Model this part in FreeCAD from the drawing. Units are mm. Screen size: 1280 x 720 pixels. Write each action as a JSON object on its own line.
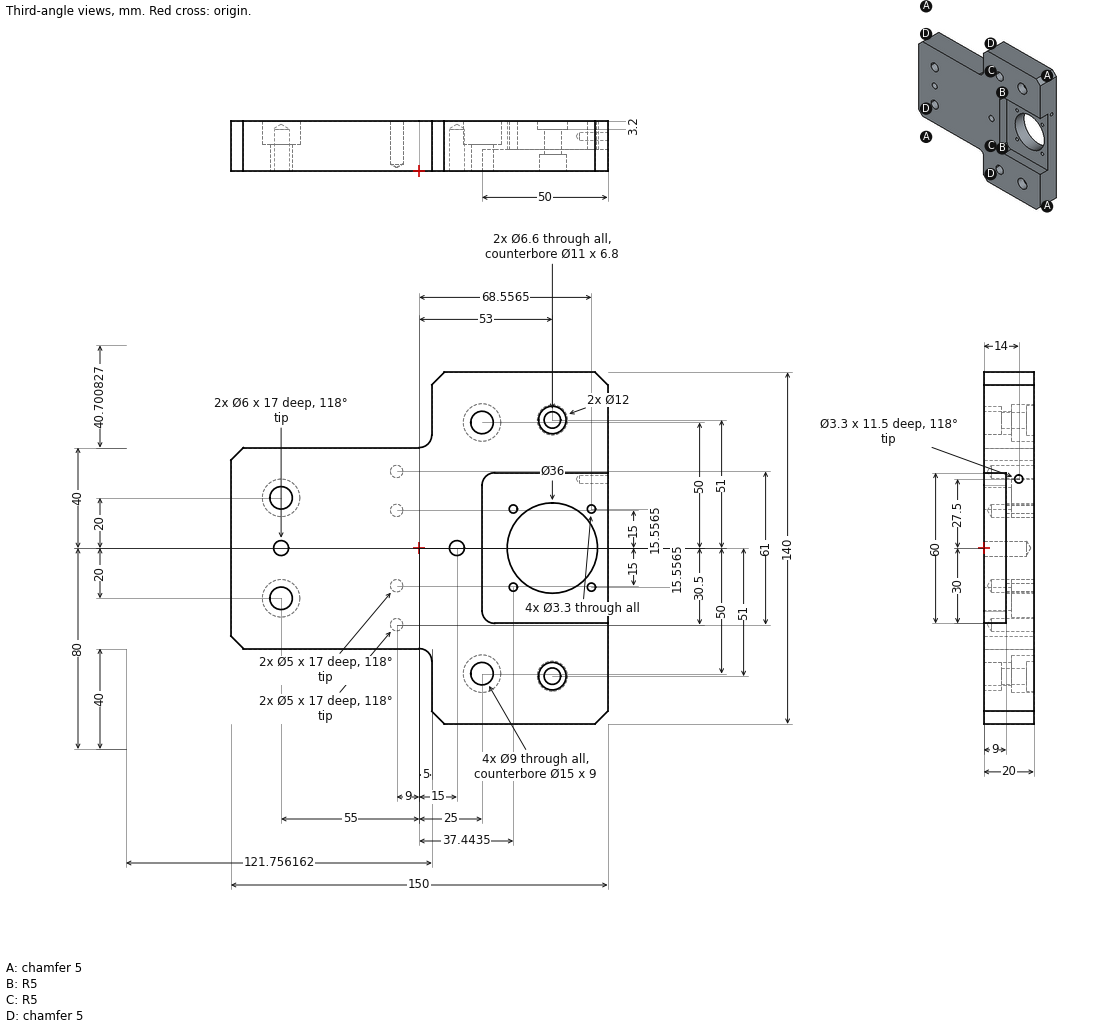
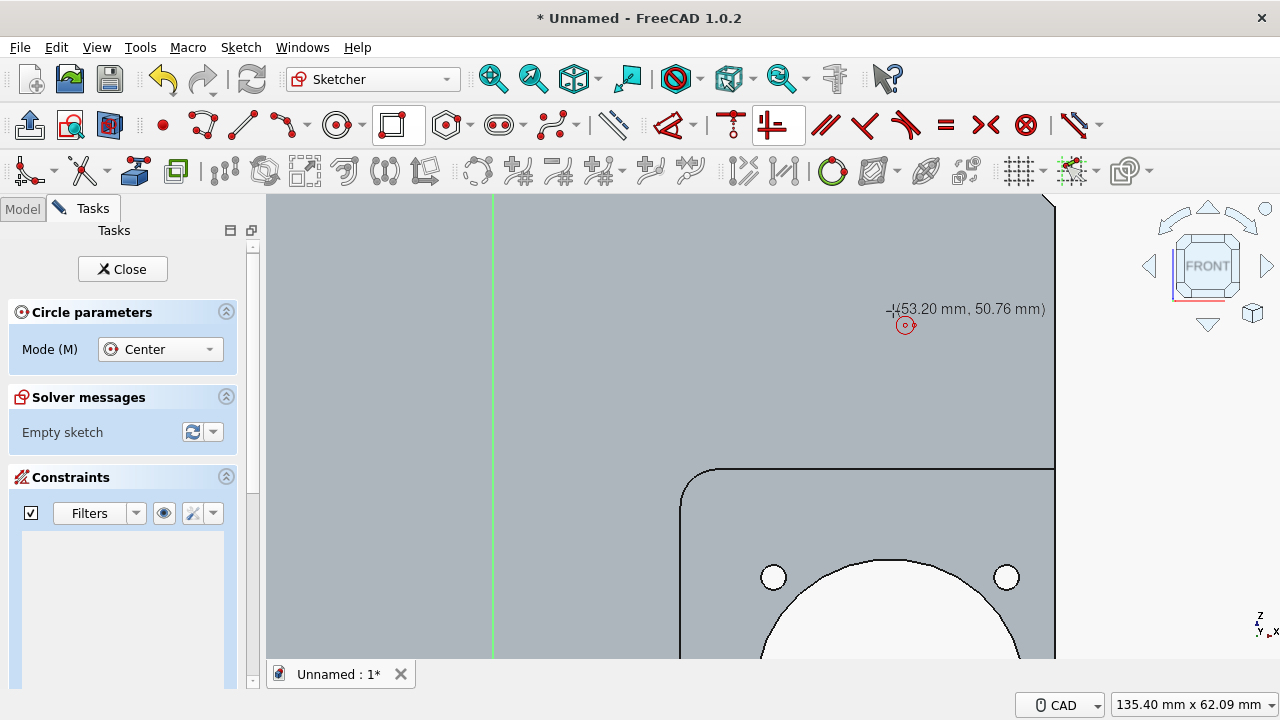
{"action": "left_click", "coordinate": [890, 312]}
{"action": "left_click", "coordinate": [908, 294]}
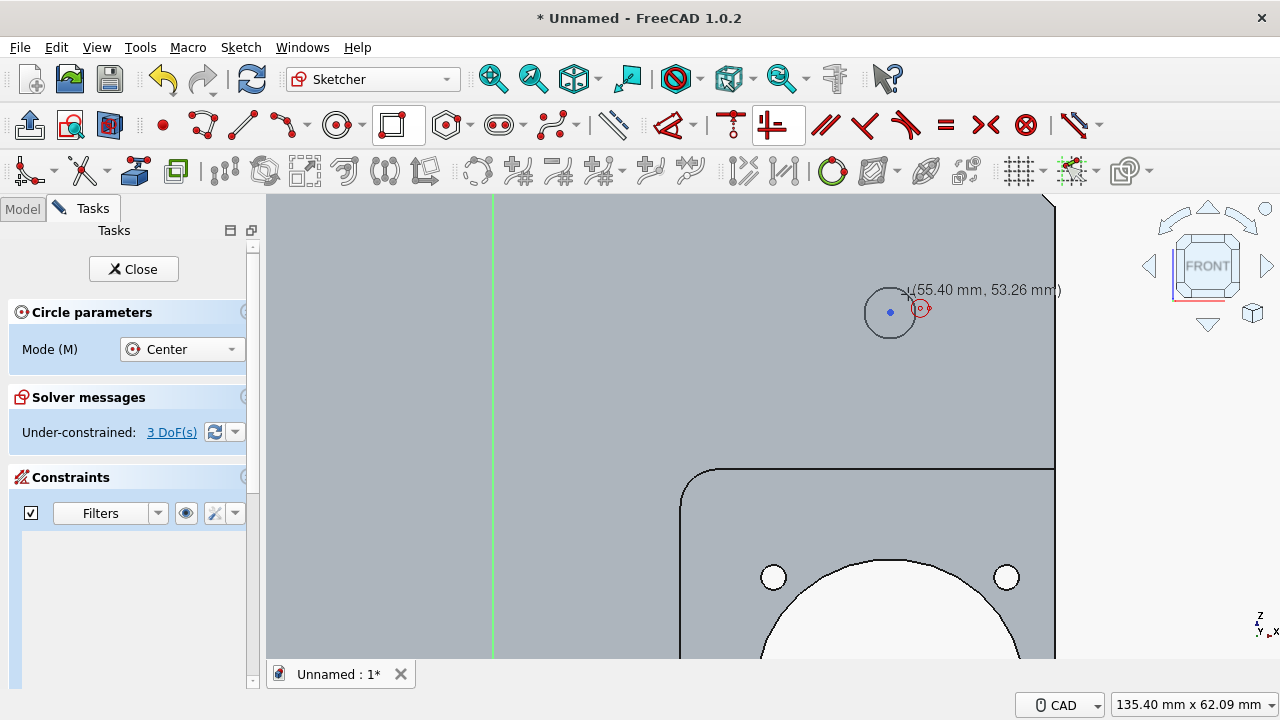
{"action": "scroll", "coordinate": [705, 271], "scroll_direction": "down", "scroll_amount": 5}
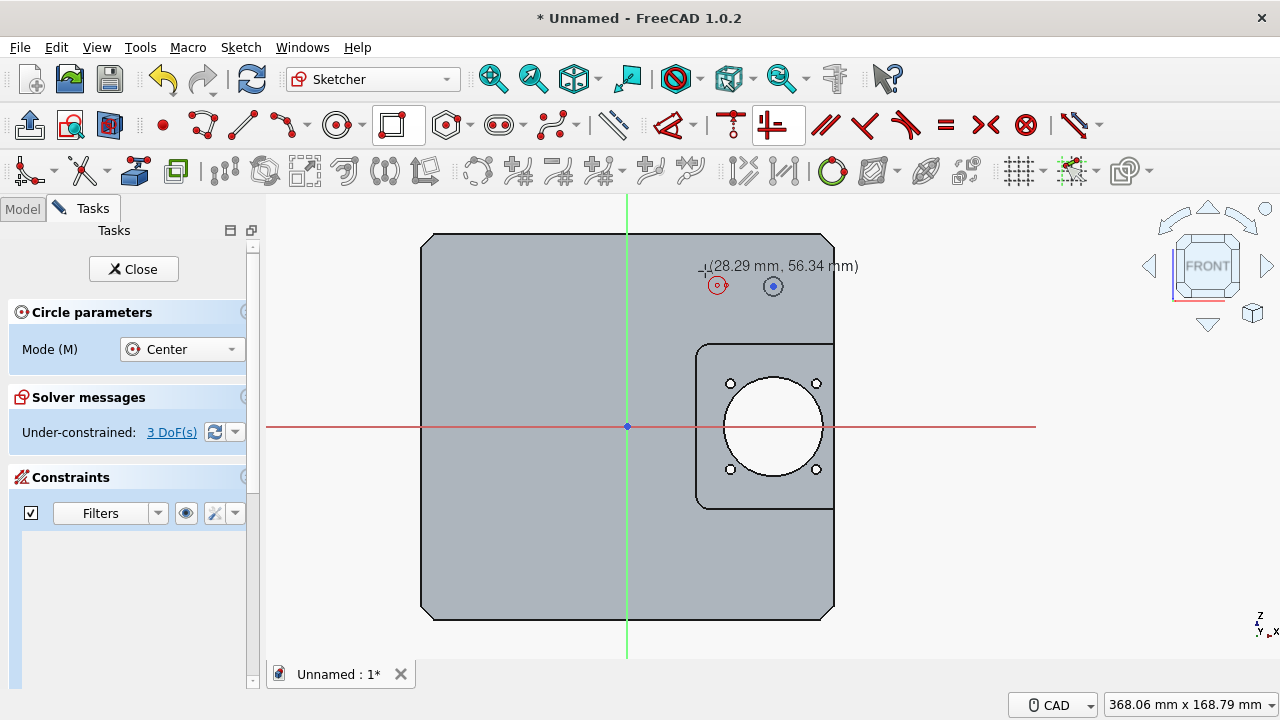
{"action": "scroll", "coordinate": [773, 567], "scroll_direction": "up", "scroll_amount": 5}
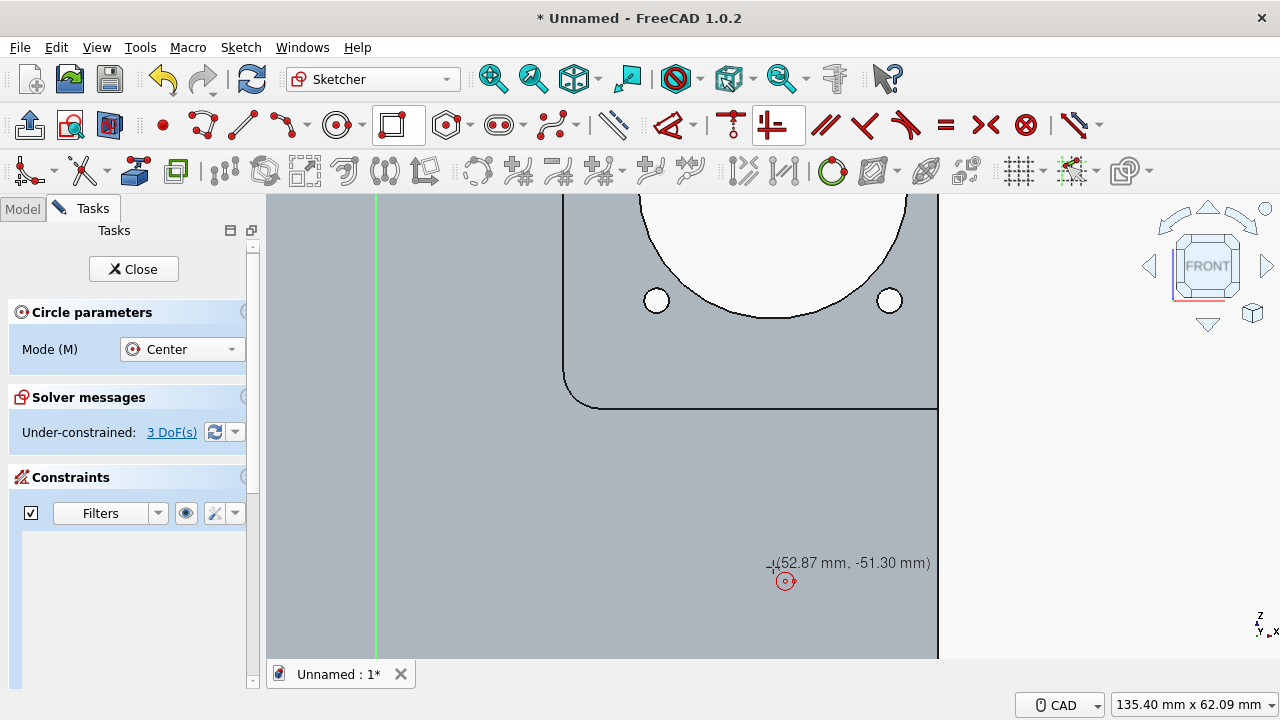
{"action": "left_click", "coordinate": [773, 566]}
{"action": "left_click", "coordinate": [791, 549]}
{"action": "key", "text": "Escape"}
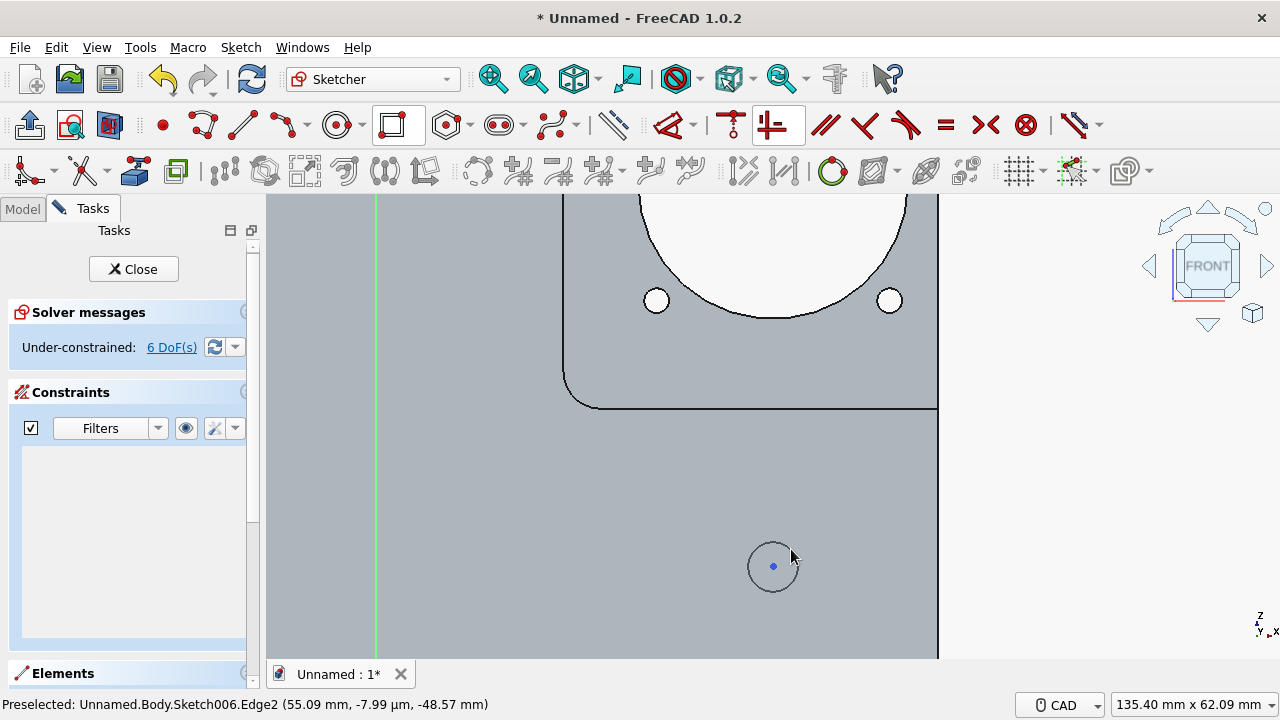
{"action": "scroll", "coordinate": [773, 568], "scroll_direction": "down", "scroll_amount": 5}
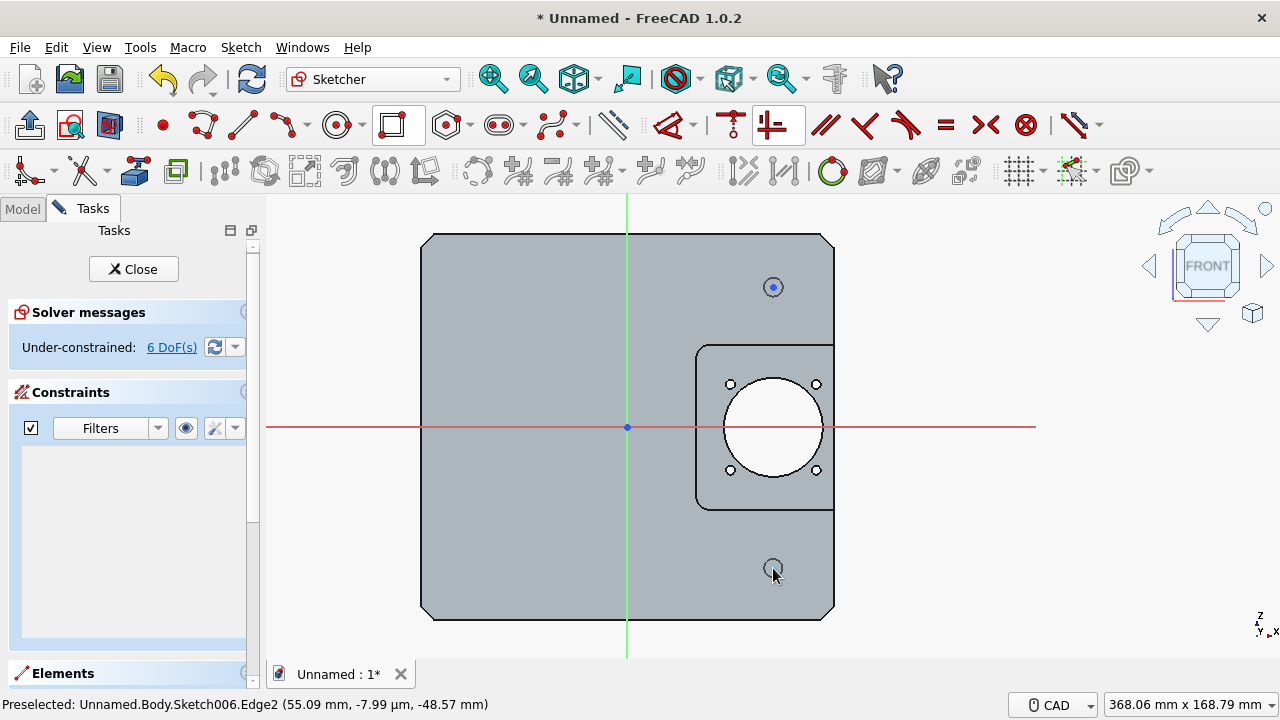
{"action": "scroll", "coordinate": [780, 281], "scroll_direction": "up", "scroll_amount": 2}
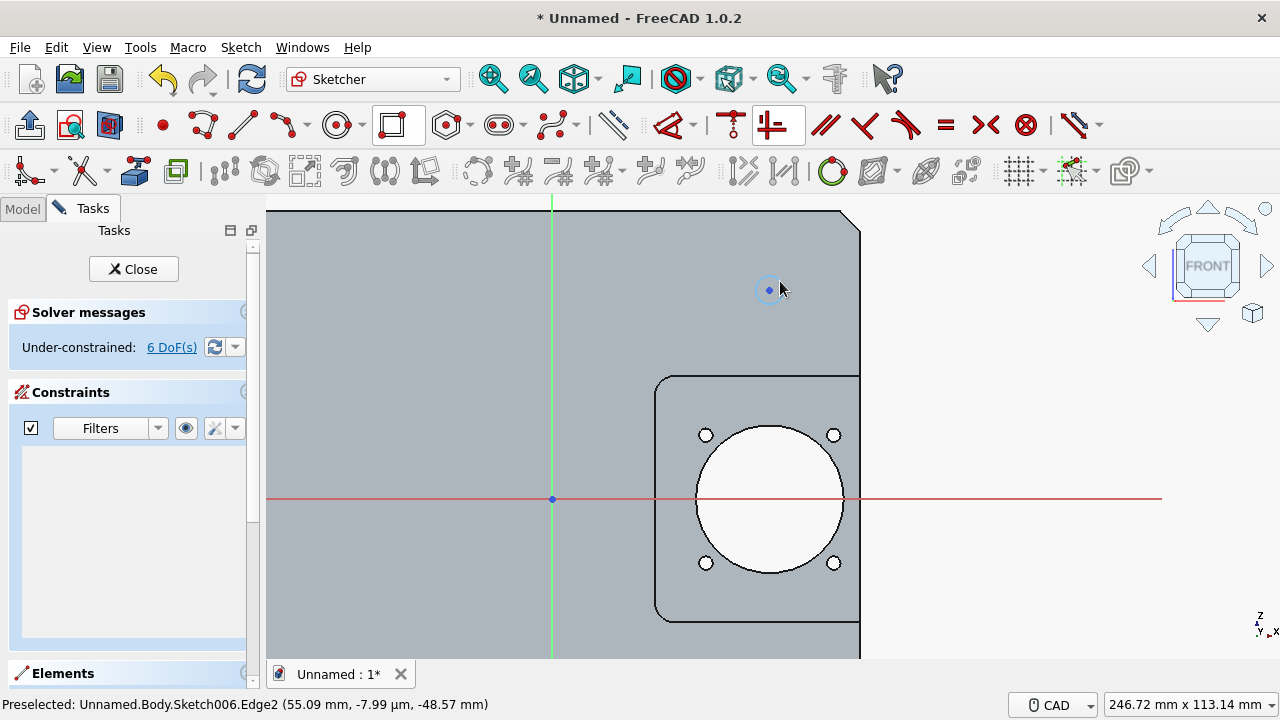
{"action": "left_click", "coordinate": [780, 280]}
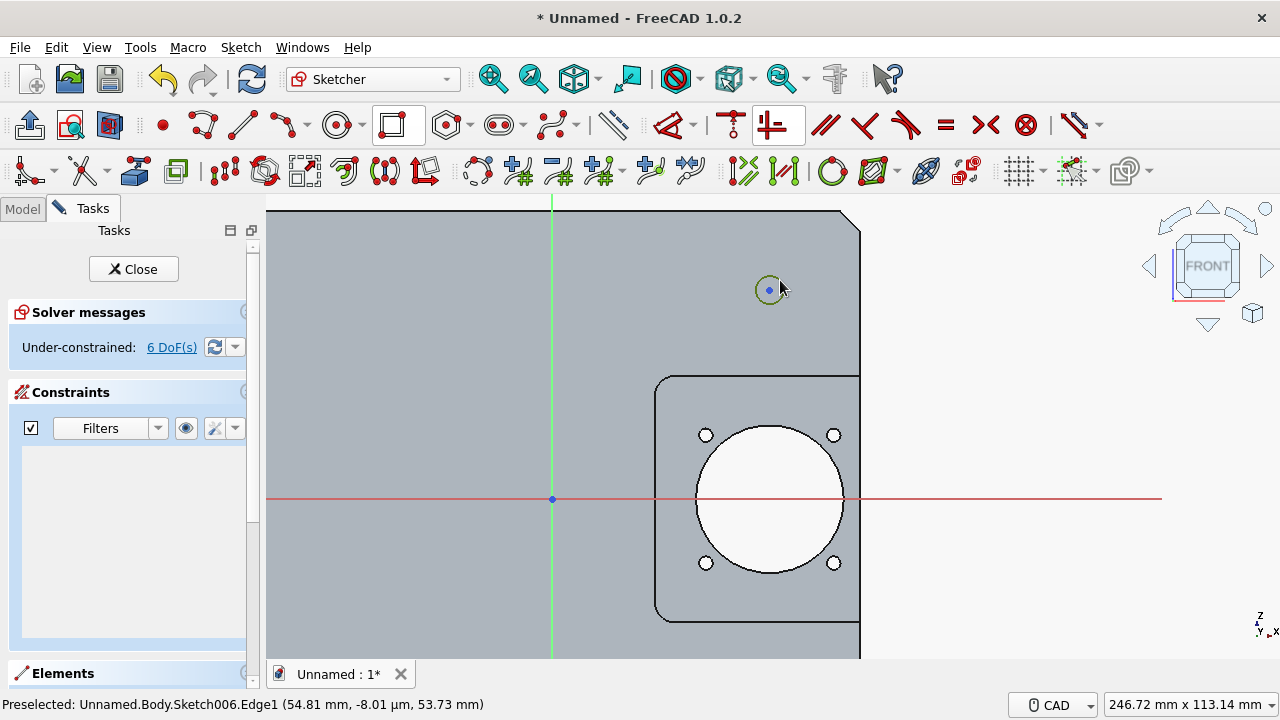
{"action": "scroll", "coordinate": [779, 279], "scroll_direction": "down", "scroll_amount": 2}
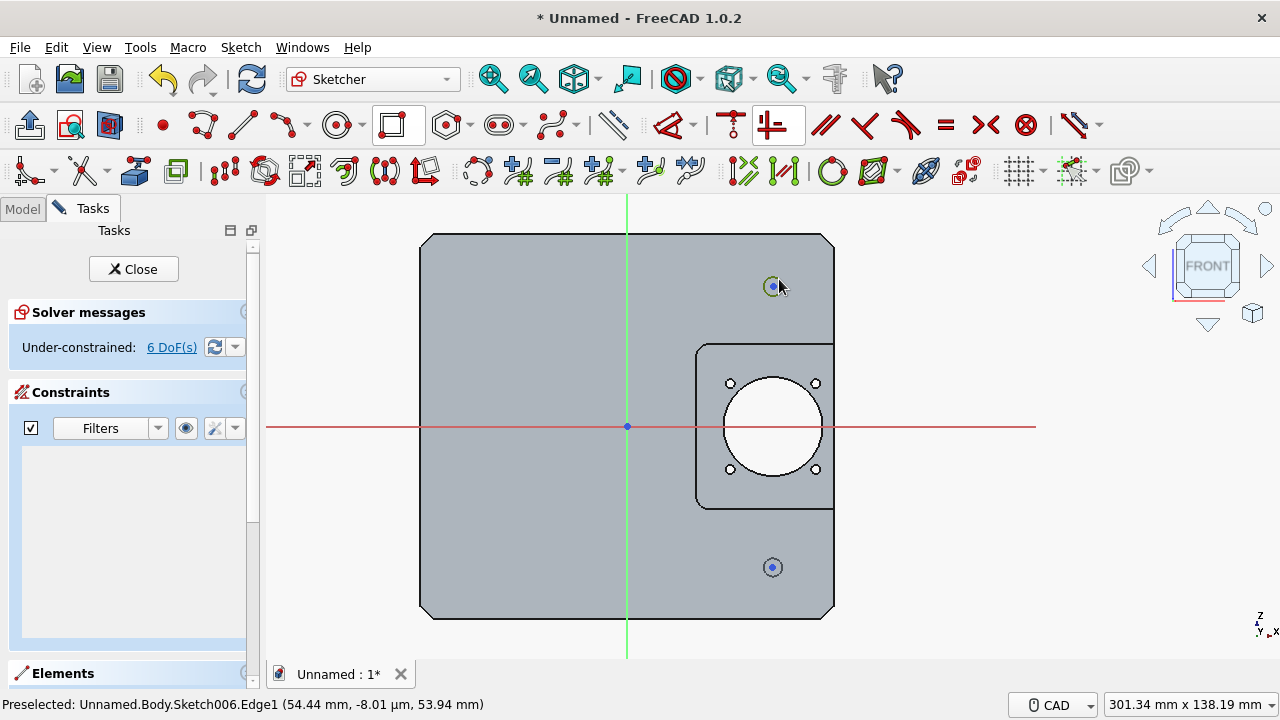
{"action": "scroll", "coordinate": [779, 561], "scroll_direction": "up", "scroll_amount": 3}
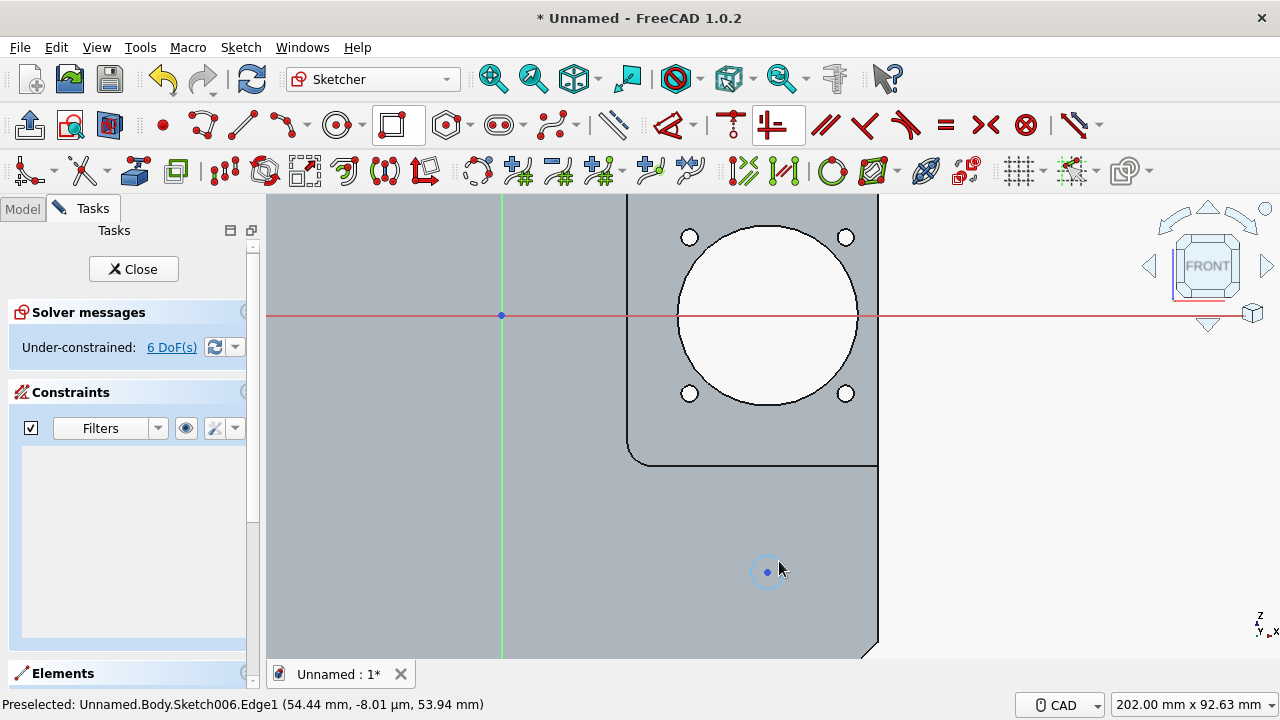
{"action": "left_click", "coordinate": [779, 560]}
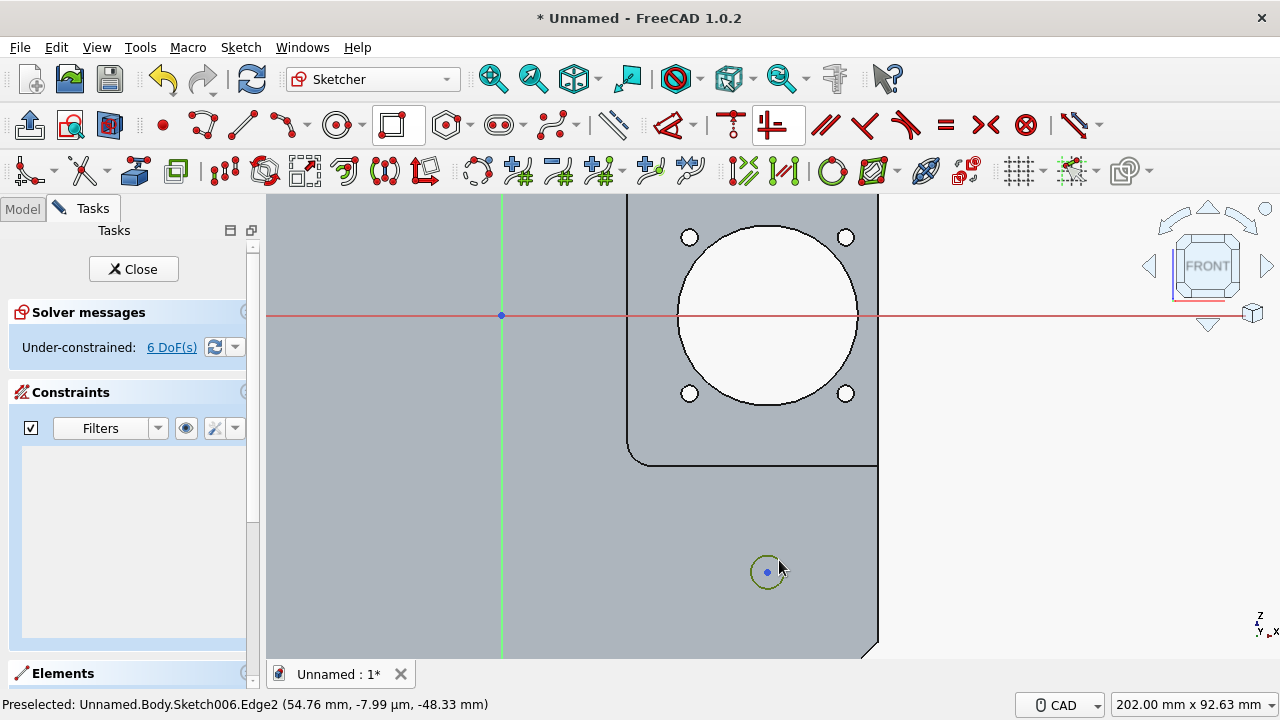
{"action": "left_click", "coordinate": [946, 126]}